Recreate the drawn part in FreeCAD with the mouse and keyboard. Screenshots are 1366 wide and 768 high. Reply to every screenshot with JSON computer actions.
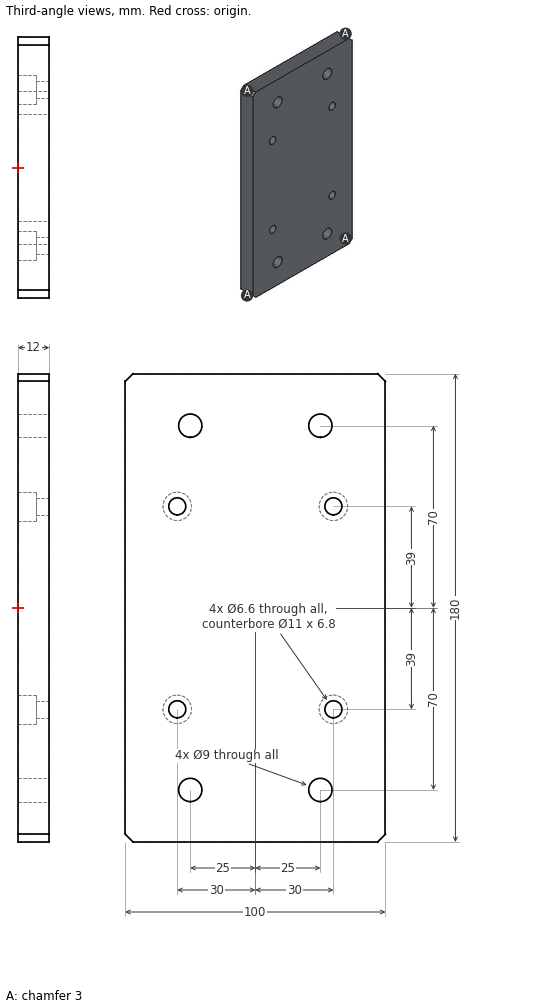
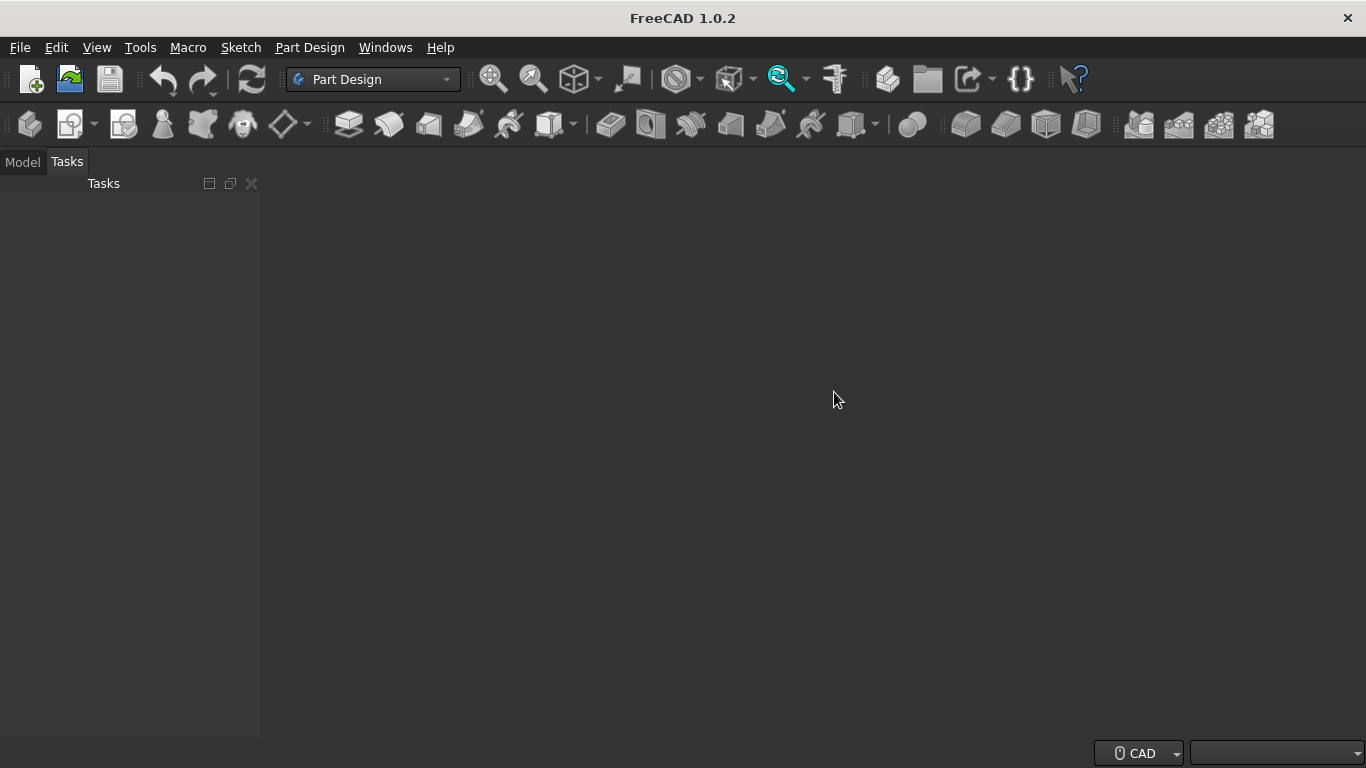
{"action": "left_click", "coordinate": [30, 80]}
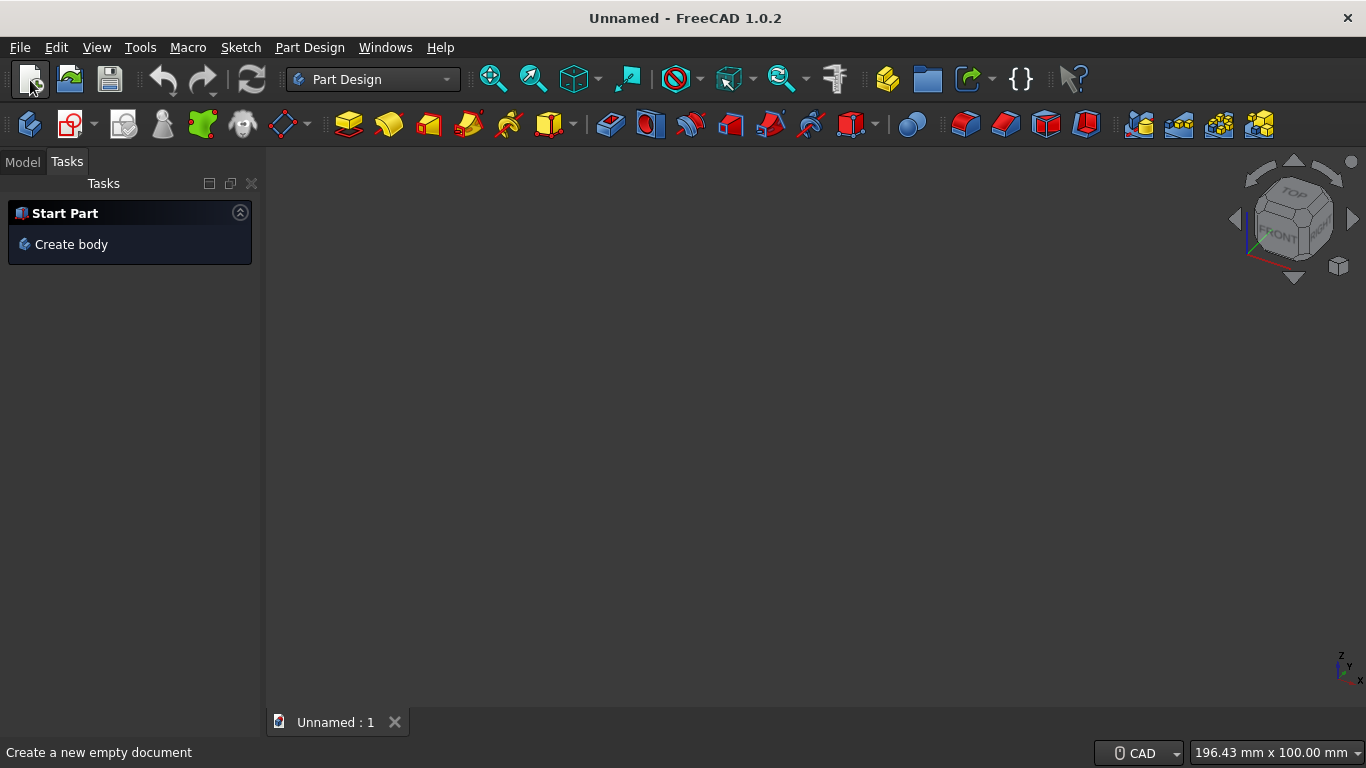
{"action": "left_click", "coordinate": [70, 124]}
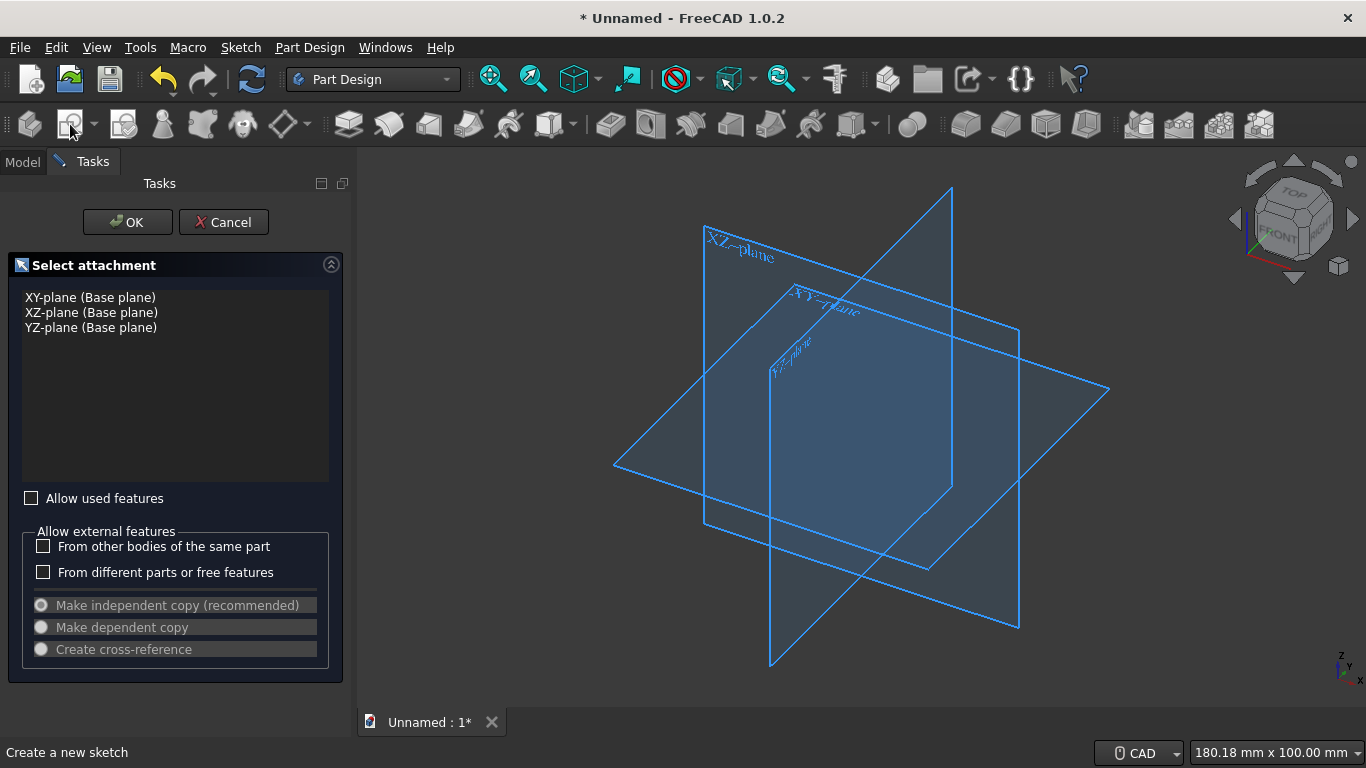
{"action": "left_click", "coordinate": [82, 328]}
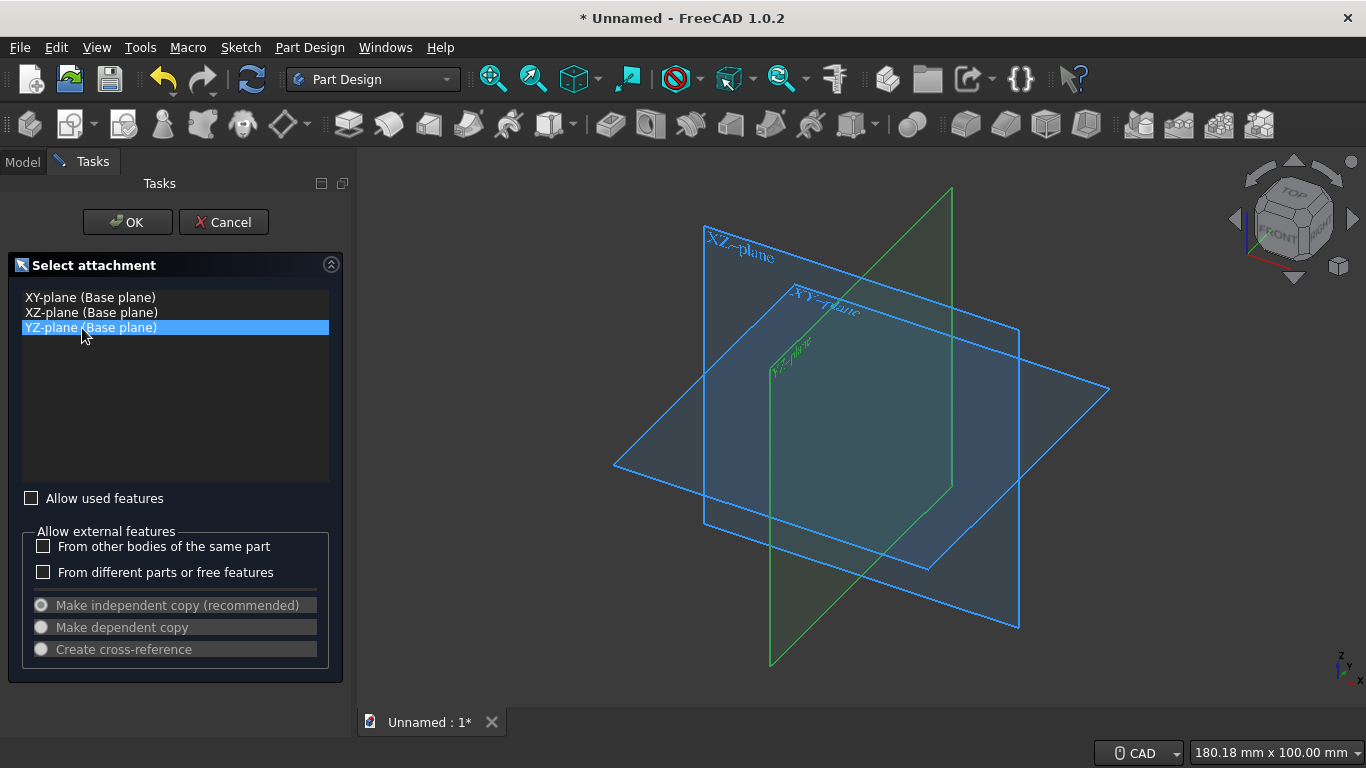
{"action": "left_click", "coordinate": [128, 222]}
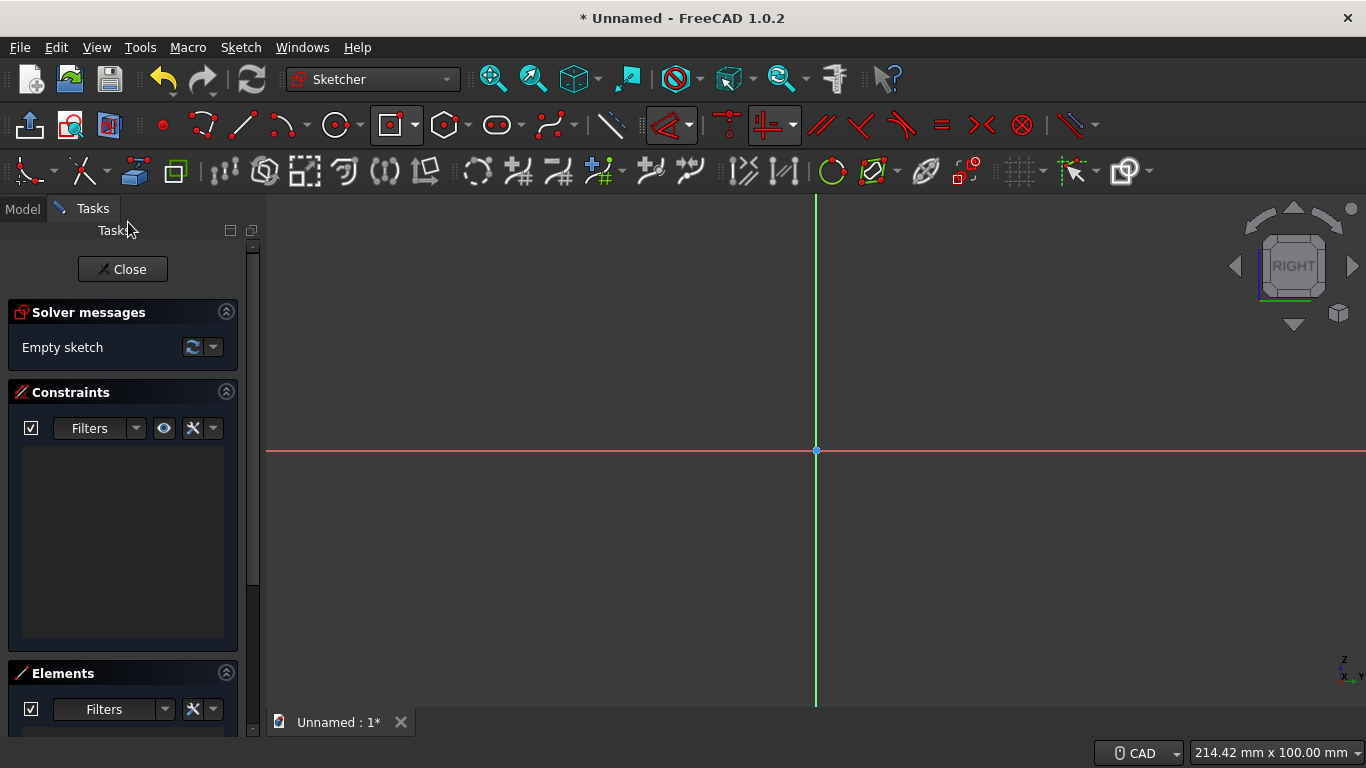
{"action": "scroll", "coordinate": [708, 450], "scroll_direction": "down", "scroll_amount": 5}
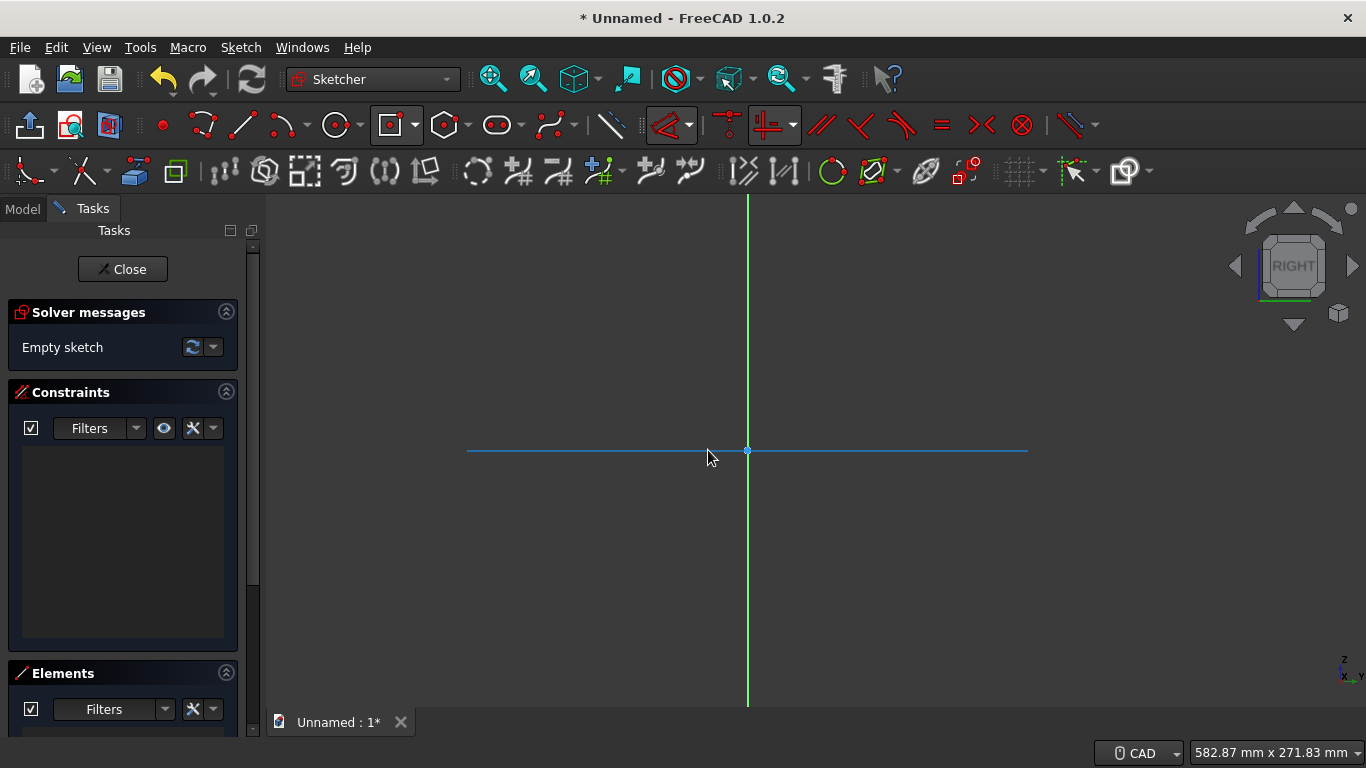
{"action": "left_click", "coordinate": [390, 126]}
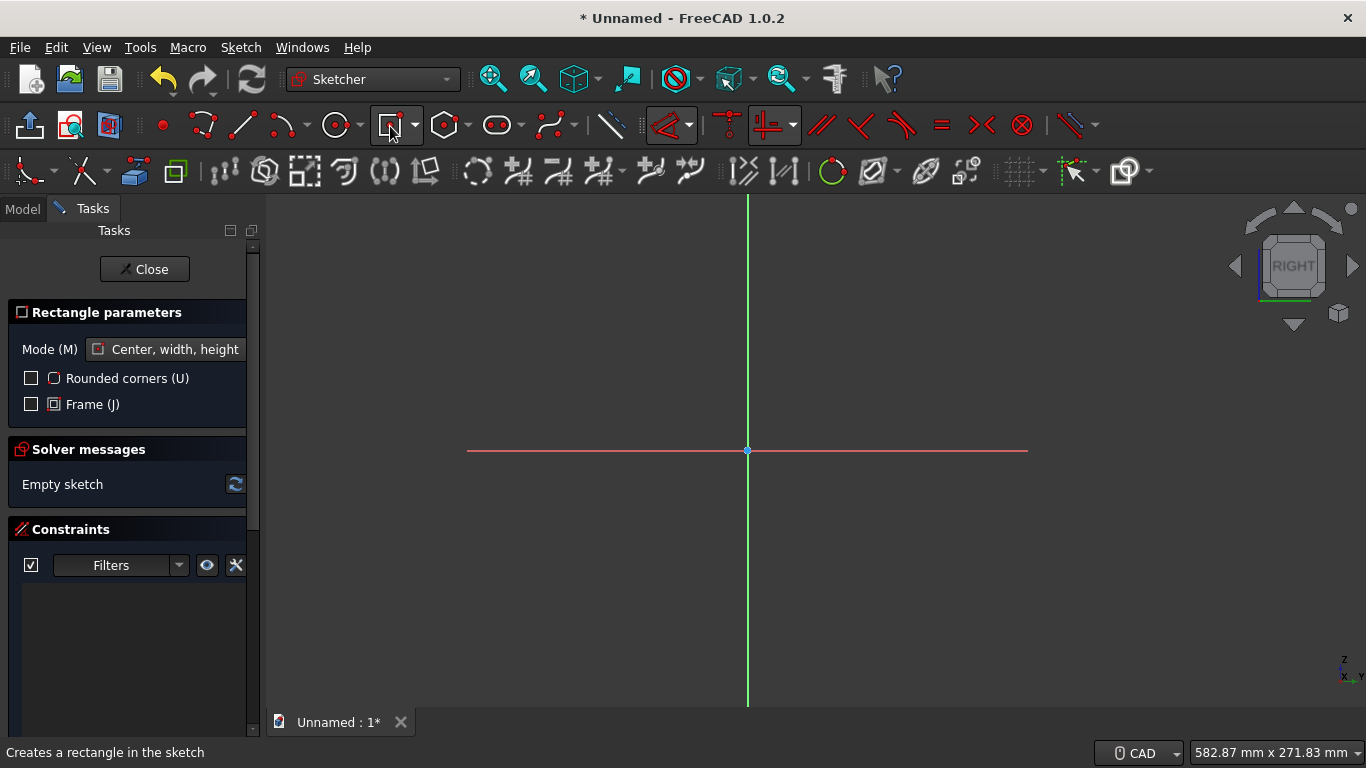
{"action": "left_click", "coordinate": [748, 450]}
{"action": "left_click", "coordinate": [842, 281]}
{"action": "key", "text": "Escape"}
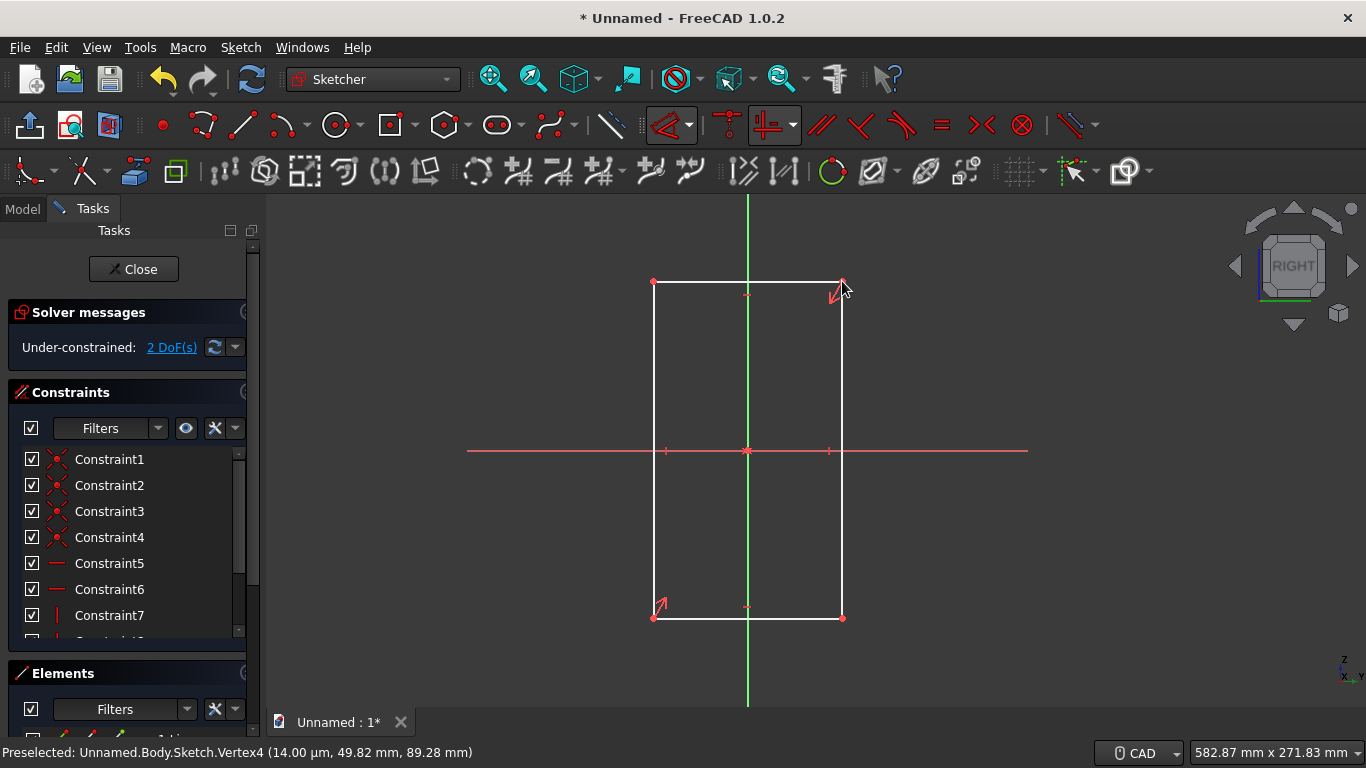
{"action": "left_click", "coordinate": [710, 619]}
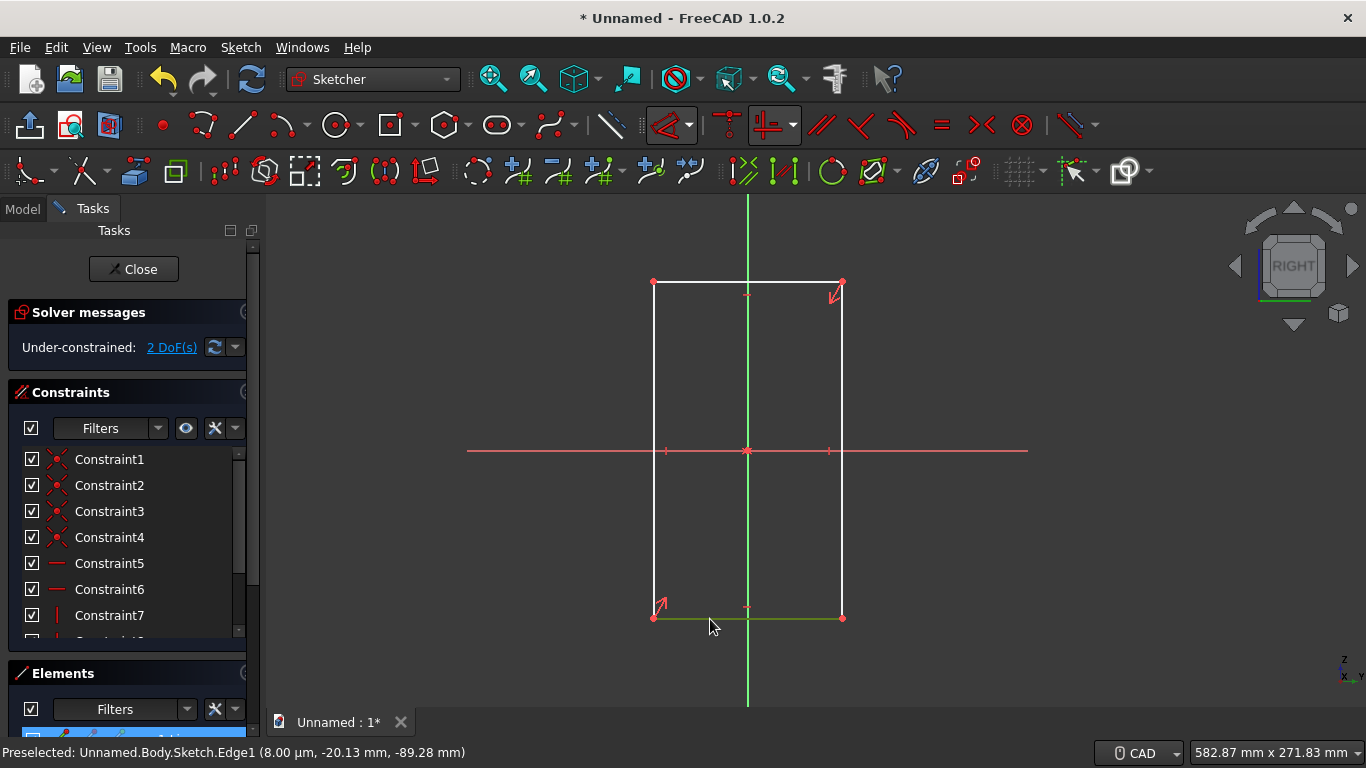
{"action": "left_click", "coordinate": [692, 126]}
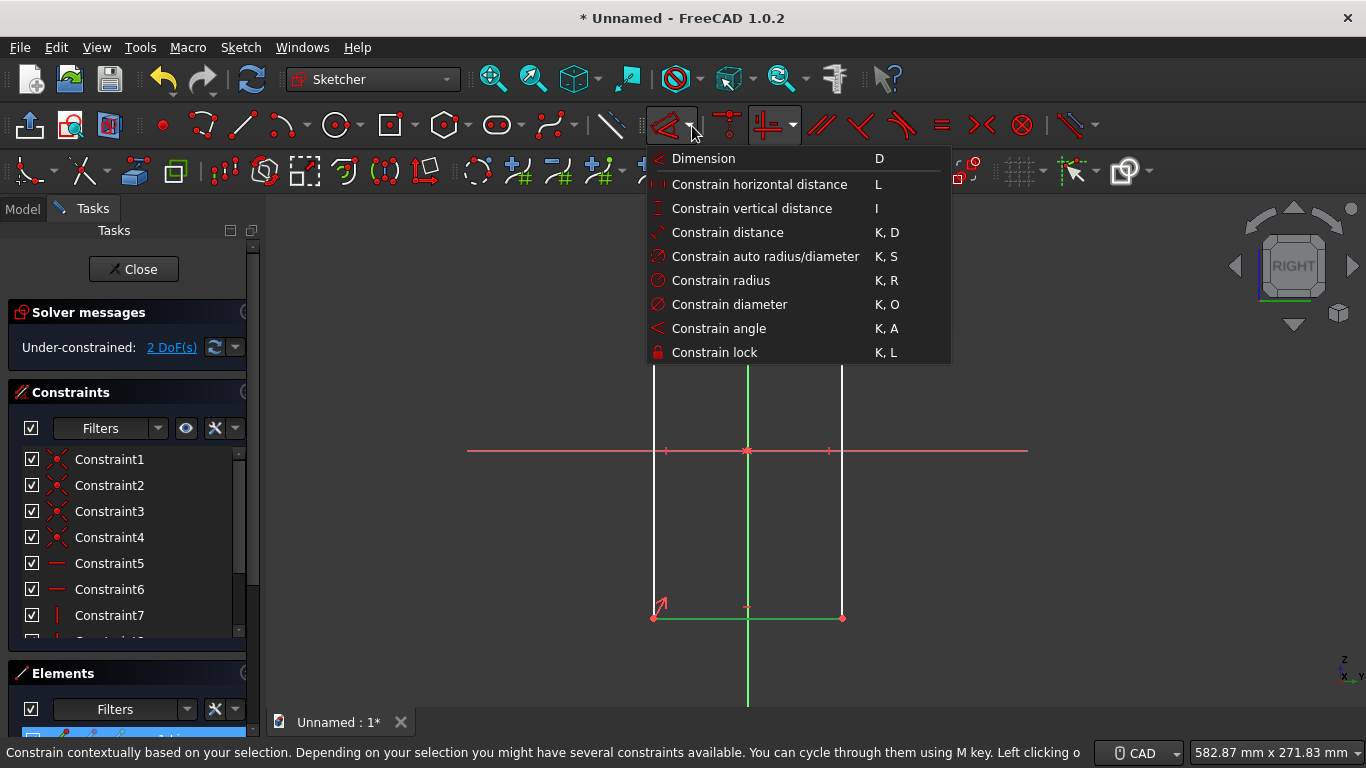
{"action": "left_click", "coordinate": [799, 184]}